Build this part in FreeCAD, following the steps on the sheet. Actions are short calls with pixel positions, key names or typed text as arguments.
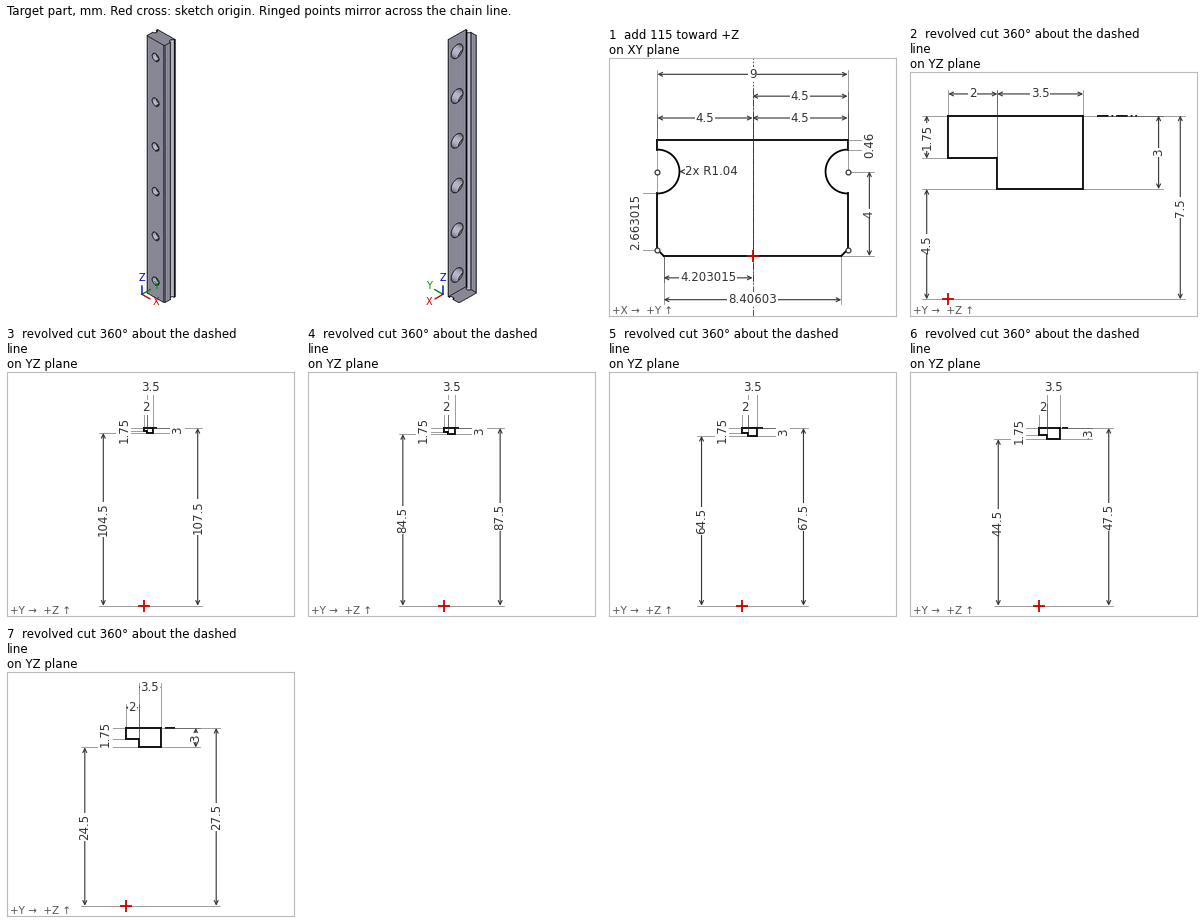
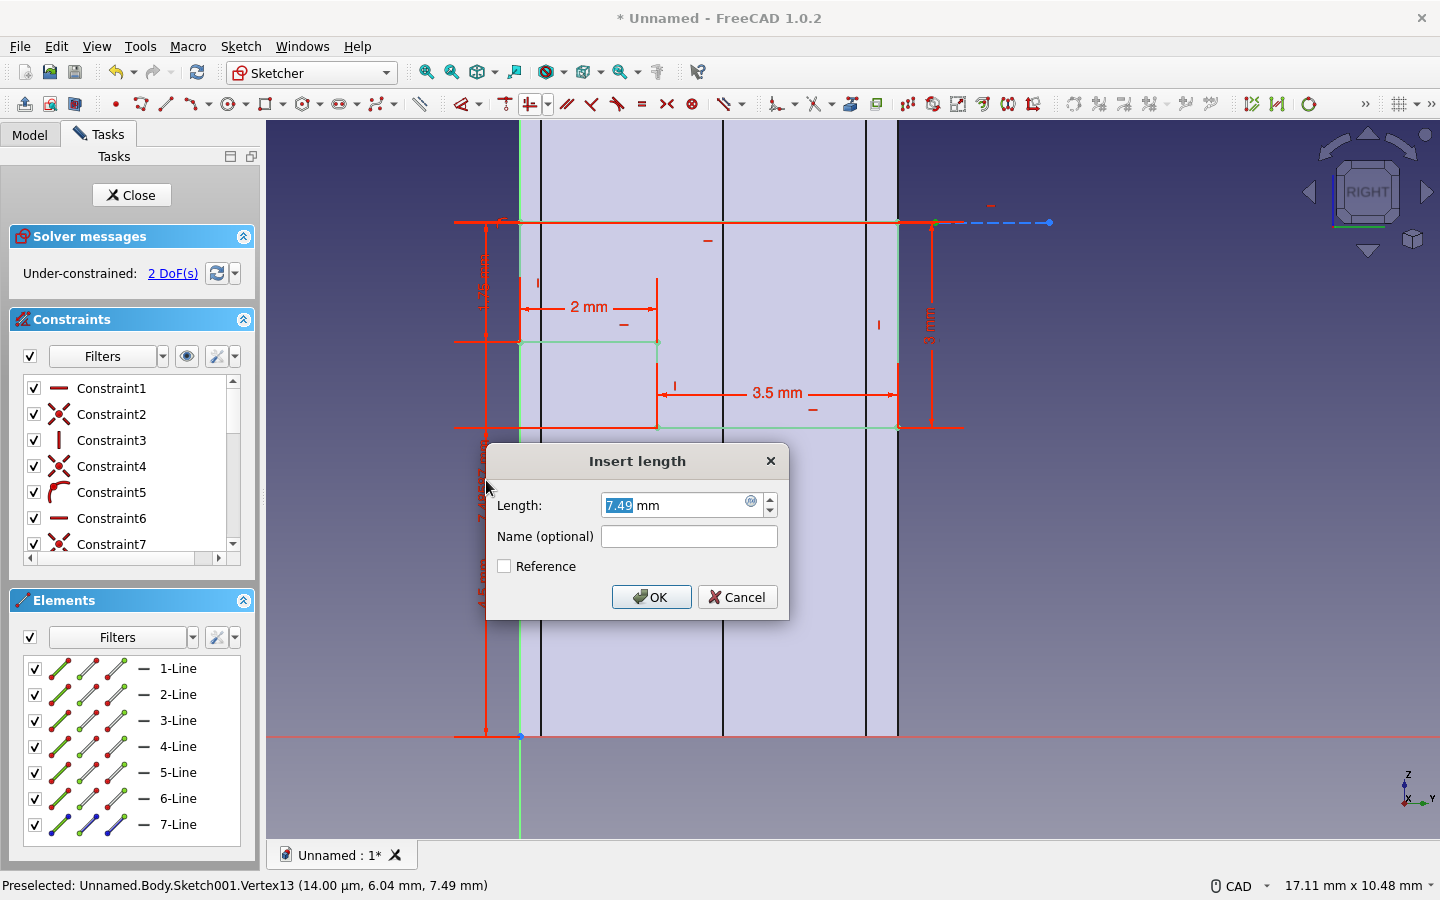
text(7.5)
key(Return)
key(Escape)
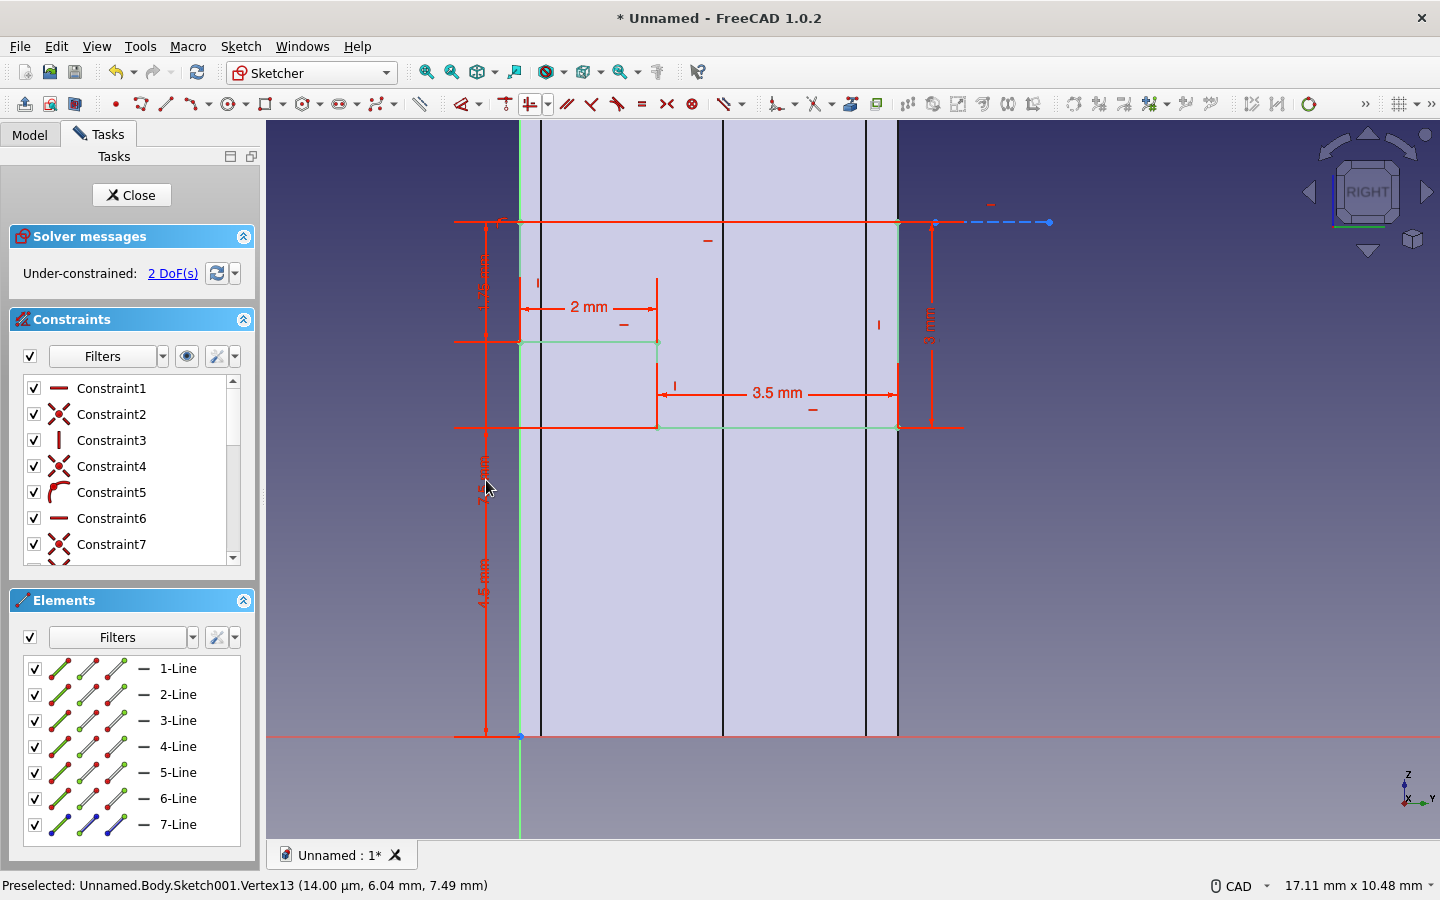
click(132, 195)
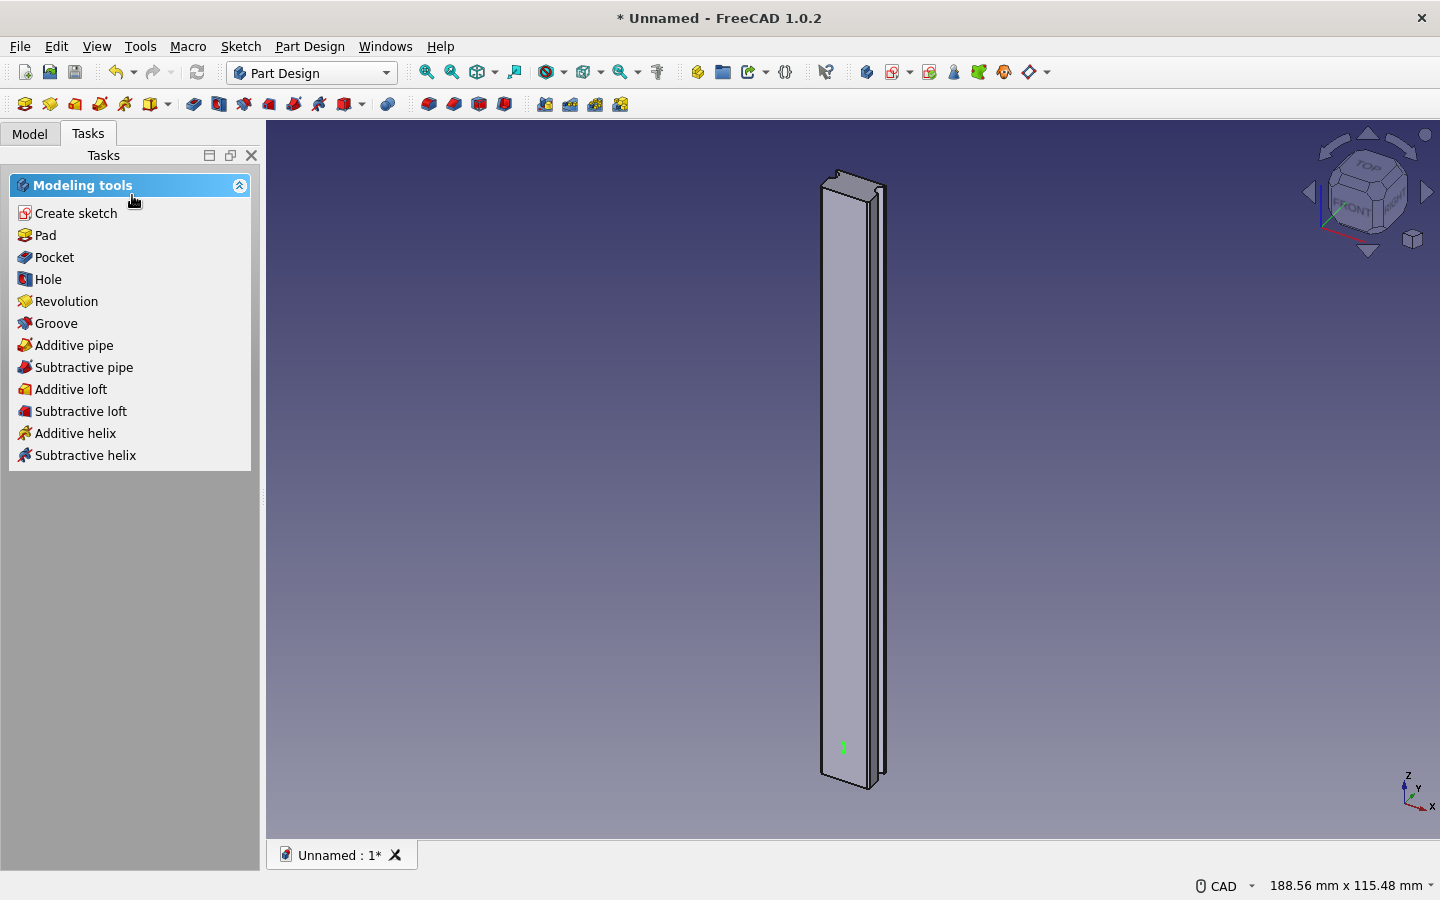
click(244, 104)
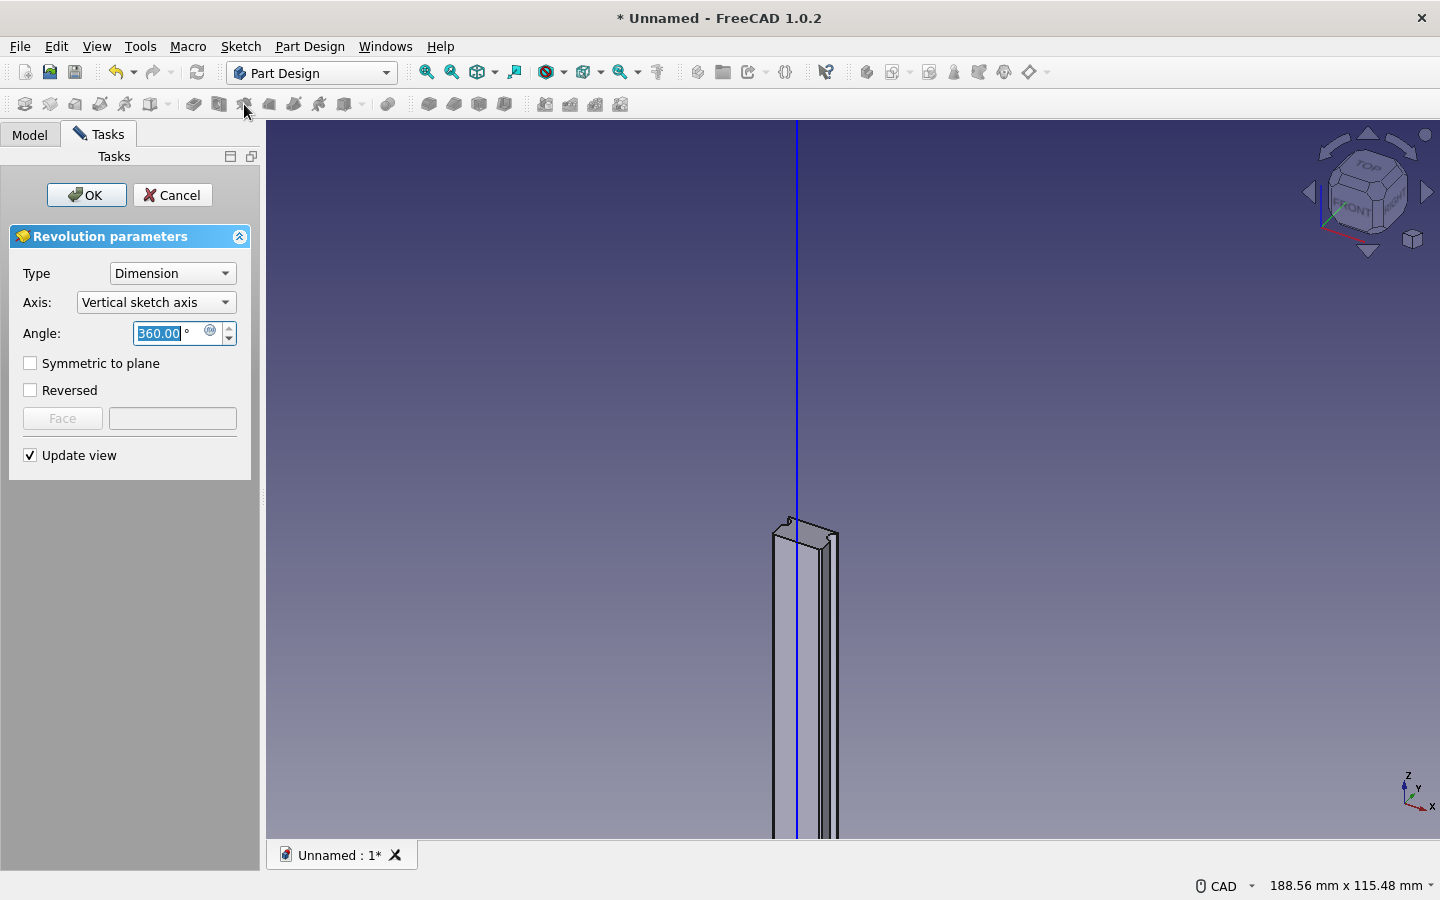
click(157, 302)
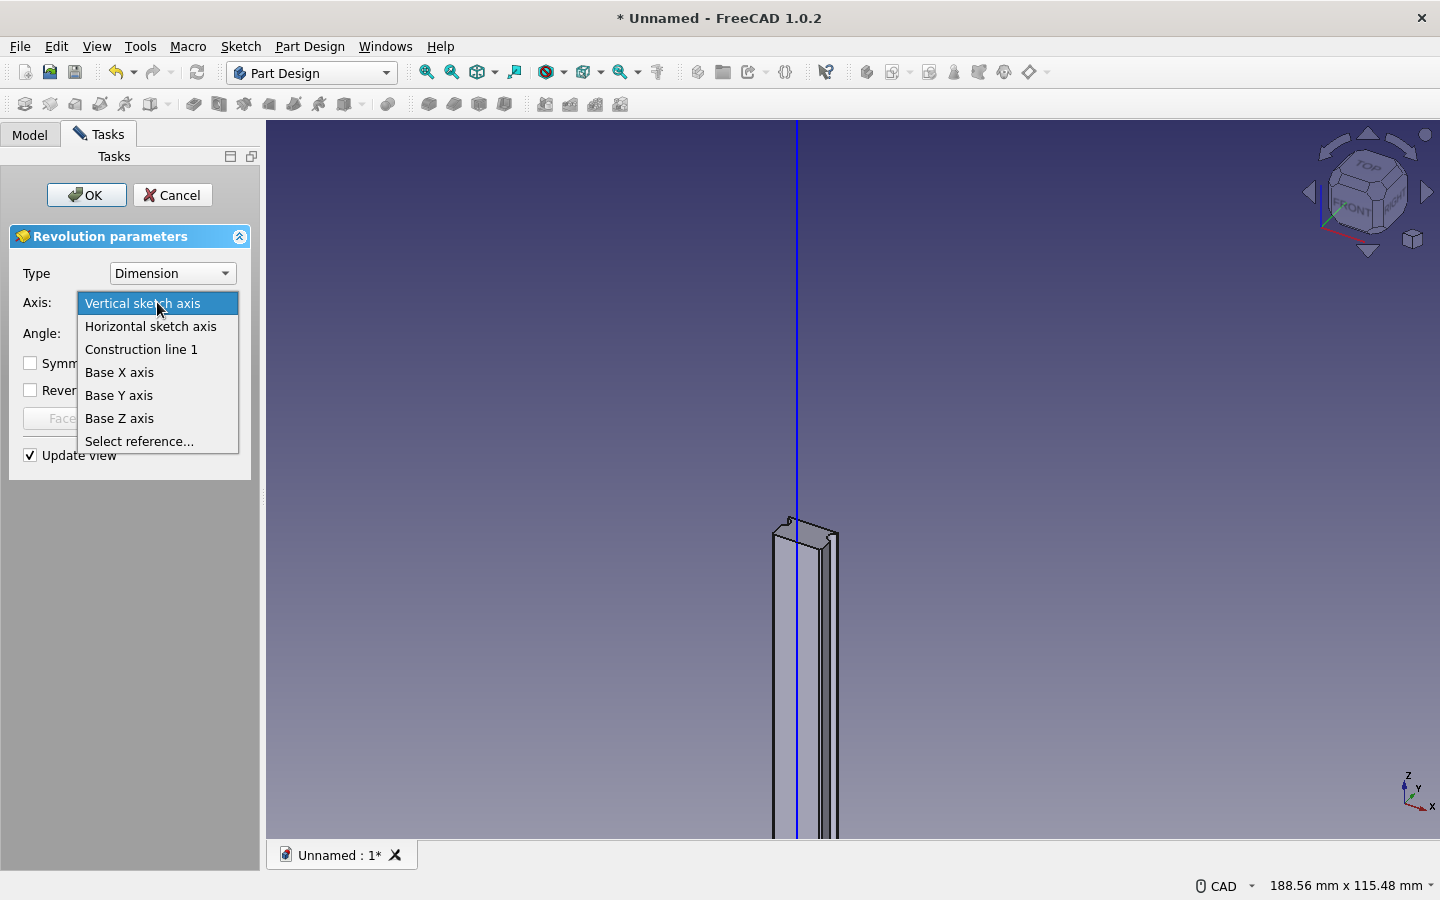
click(156, 350)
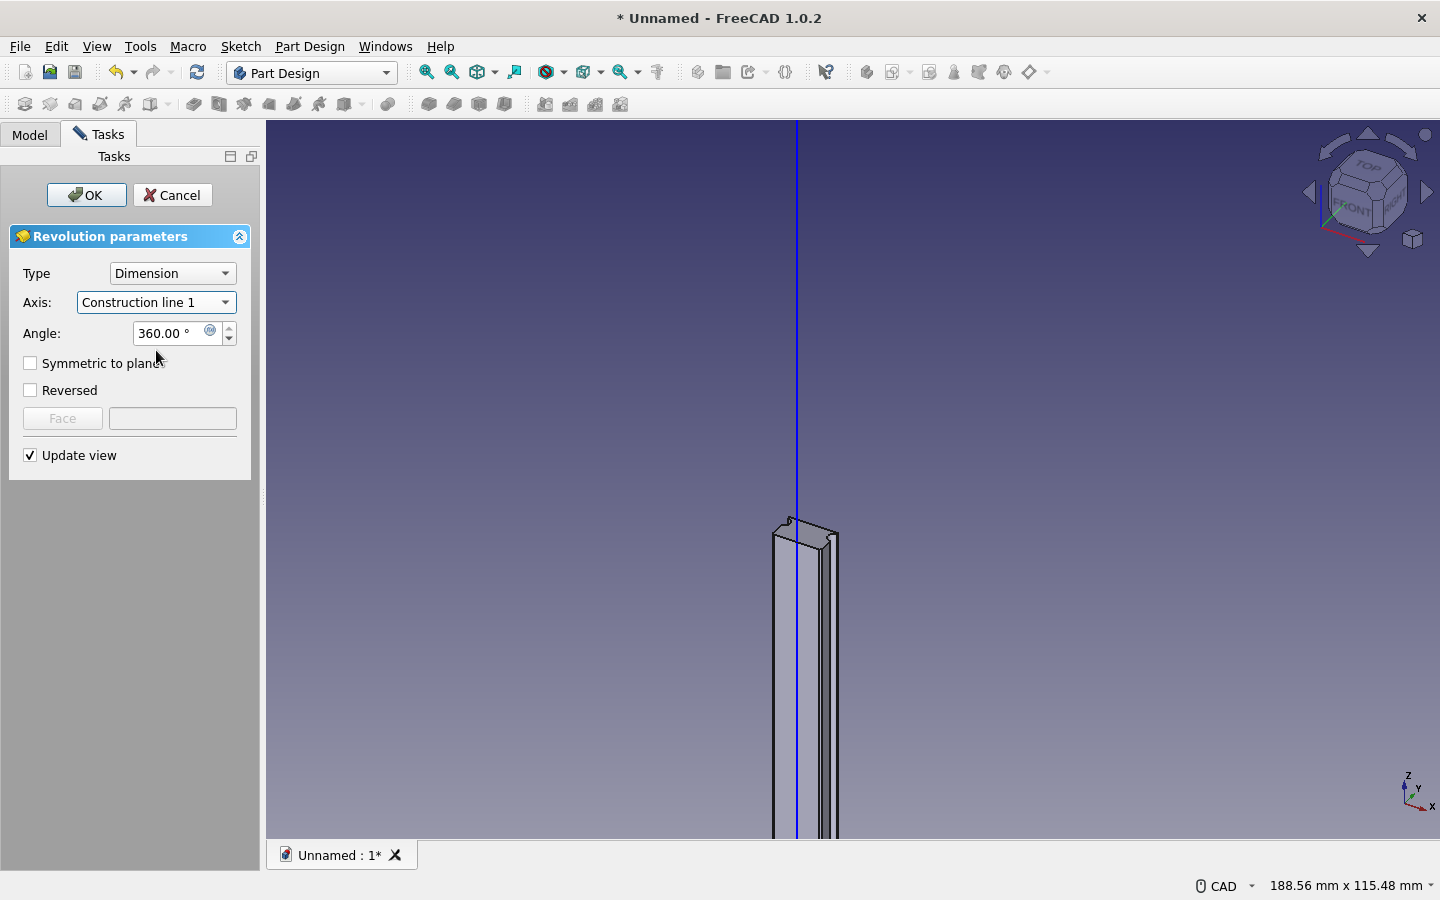
click(87, 195)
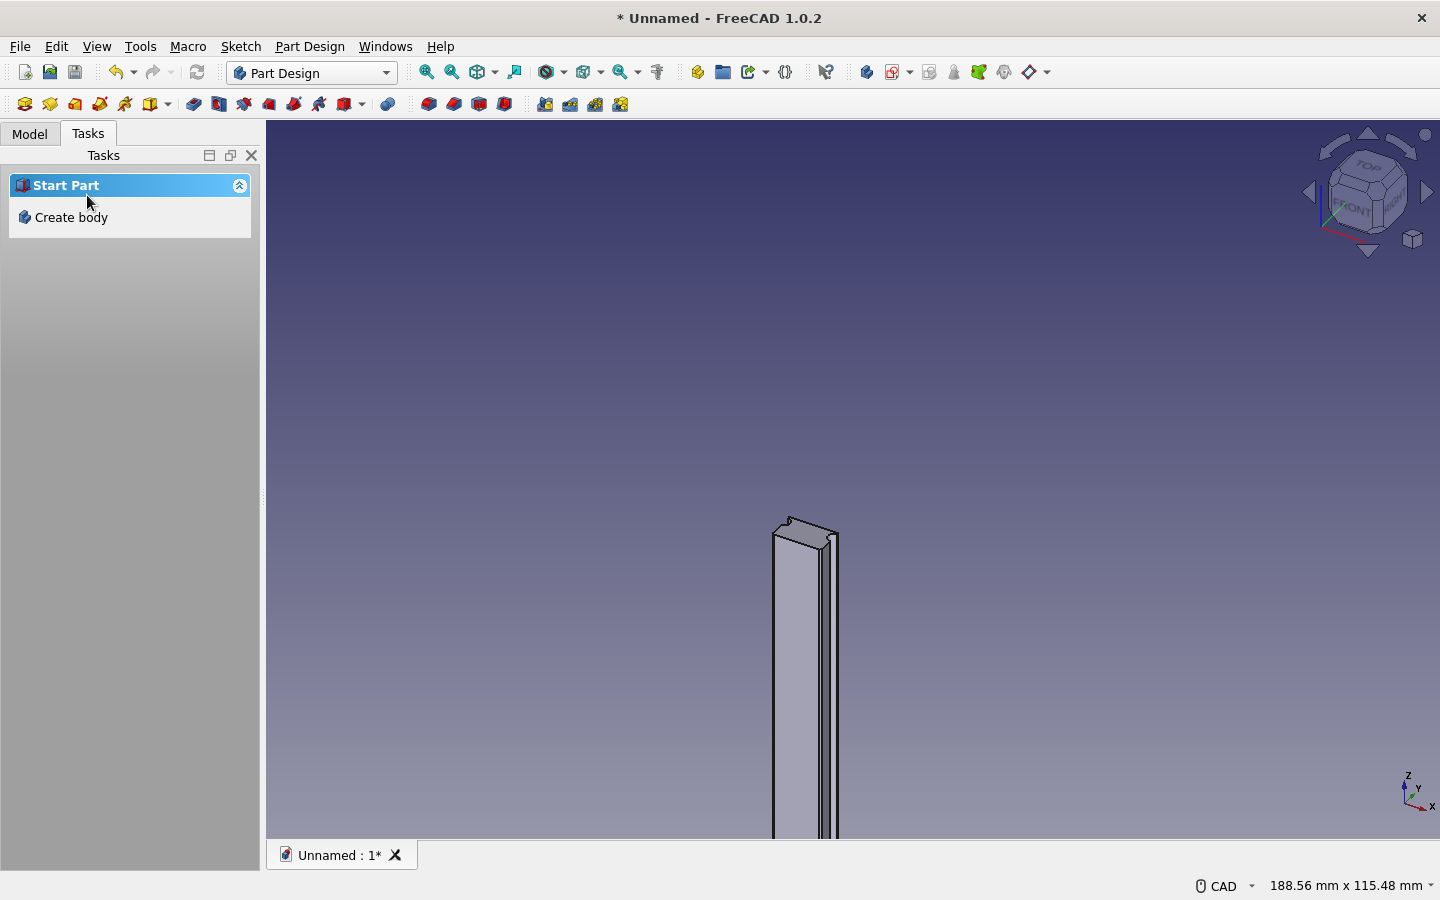
key(v)
key(f)